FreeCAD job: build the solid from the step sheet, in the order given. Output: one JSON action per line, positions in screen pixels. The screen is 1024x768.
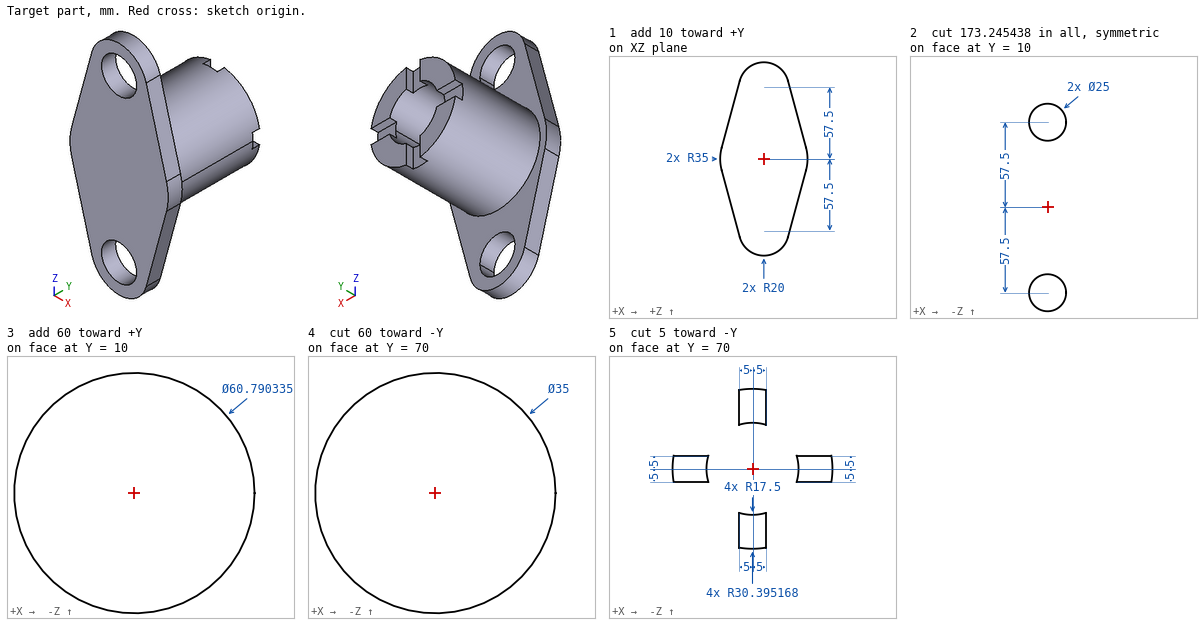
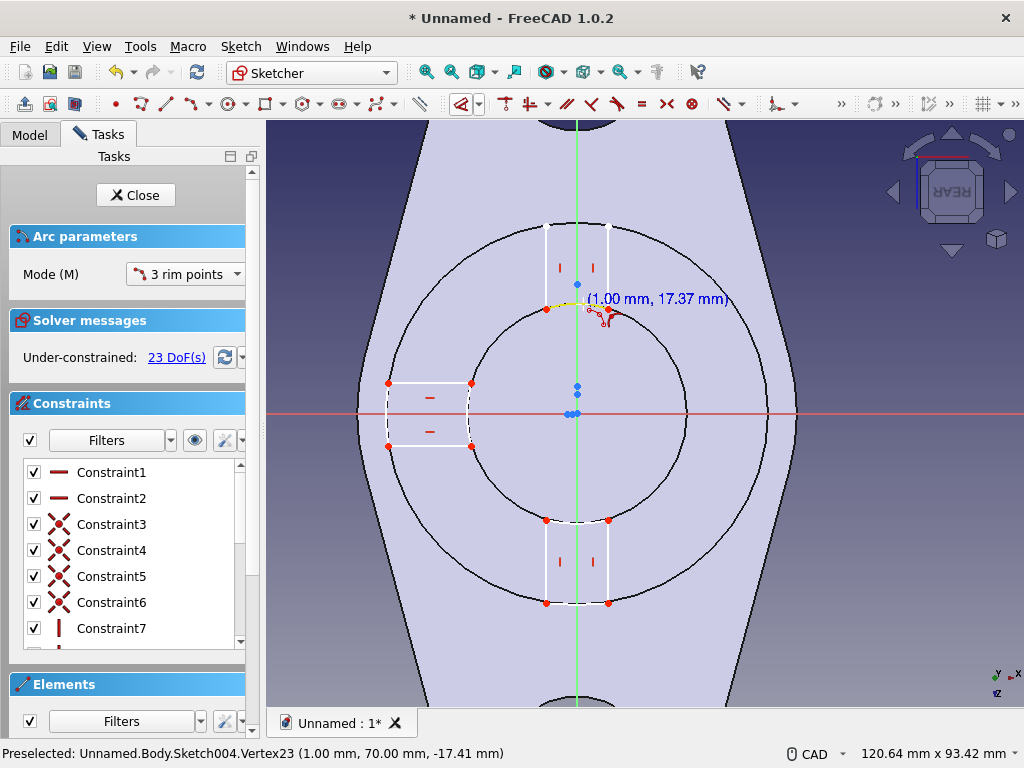
{"action": "left_click", "coordinate": [608, 226]}
{"action": "left_click", "coordinate": [546, 226]}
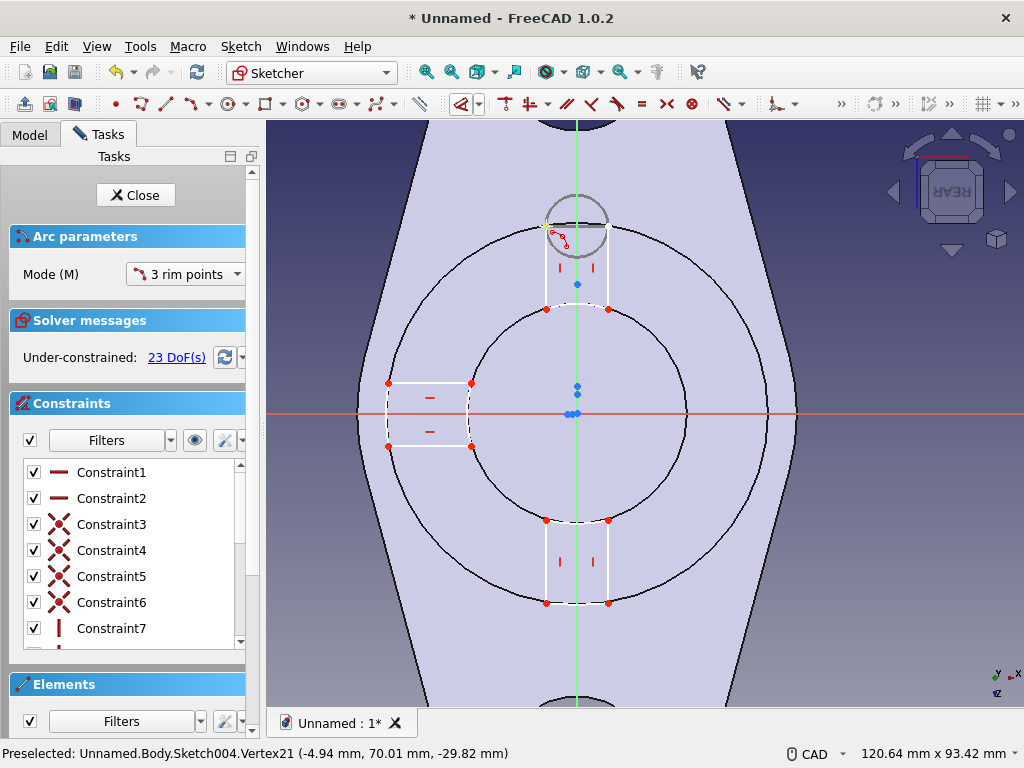
{"action": "scroll", "coordinate": [583, 223], "scroll_direction": "up", "scroll_amount": 10}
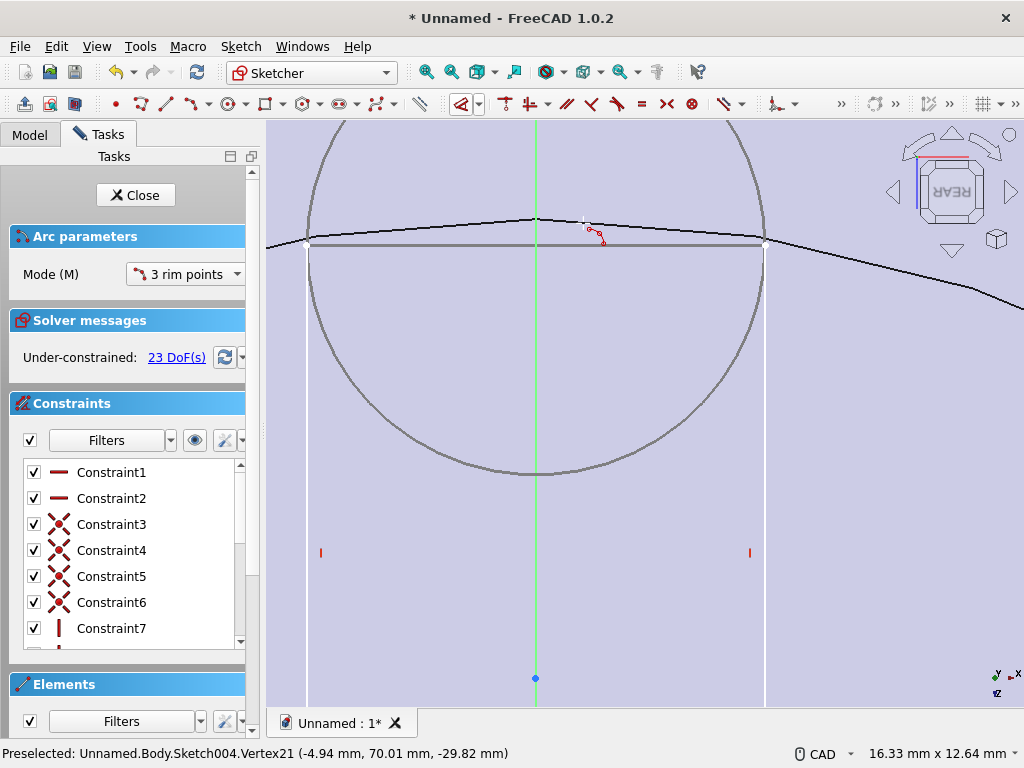
{"action": "left_click", "coordinate": [583, 220]}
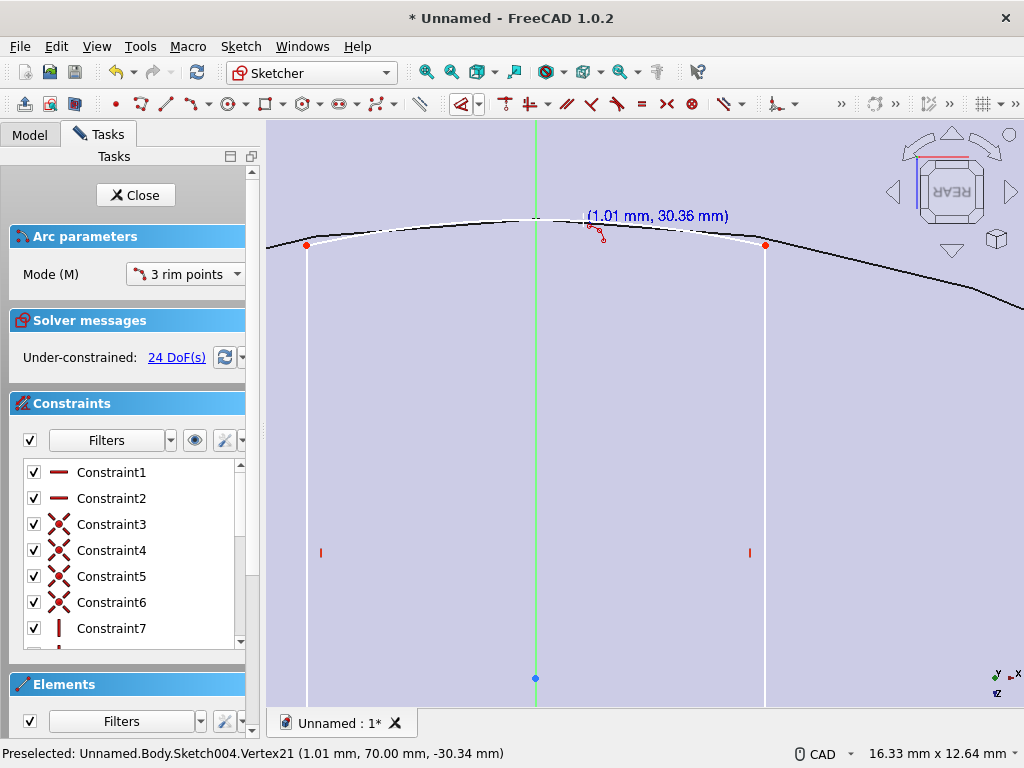
{"action": "key", "text": "g l"}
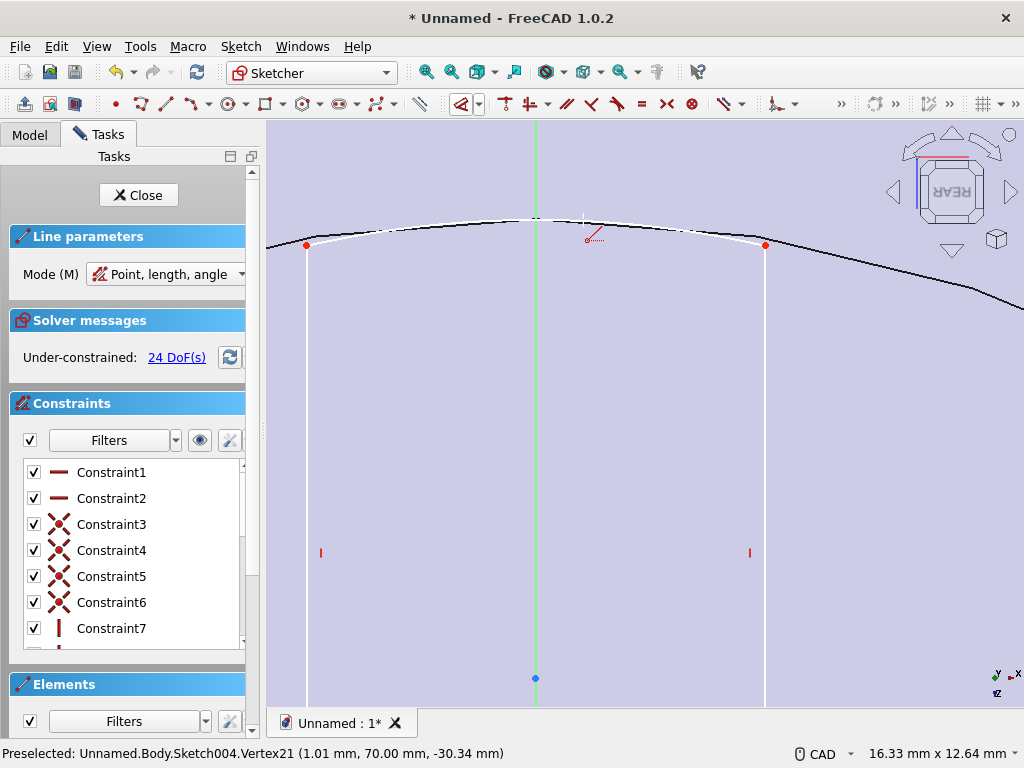
{"action": "scroll", "coordinate": [583, 223], "scroll_direction": "down", "scroll_amount": 10}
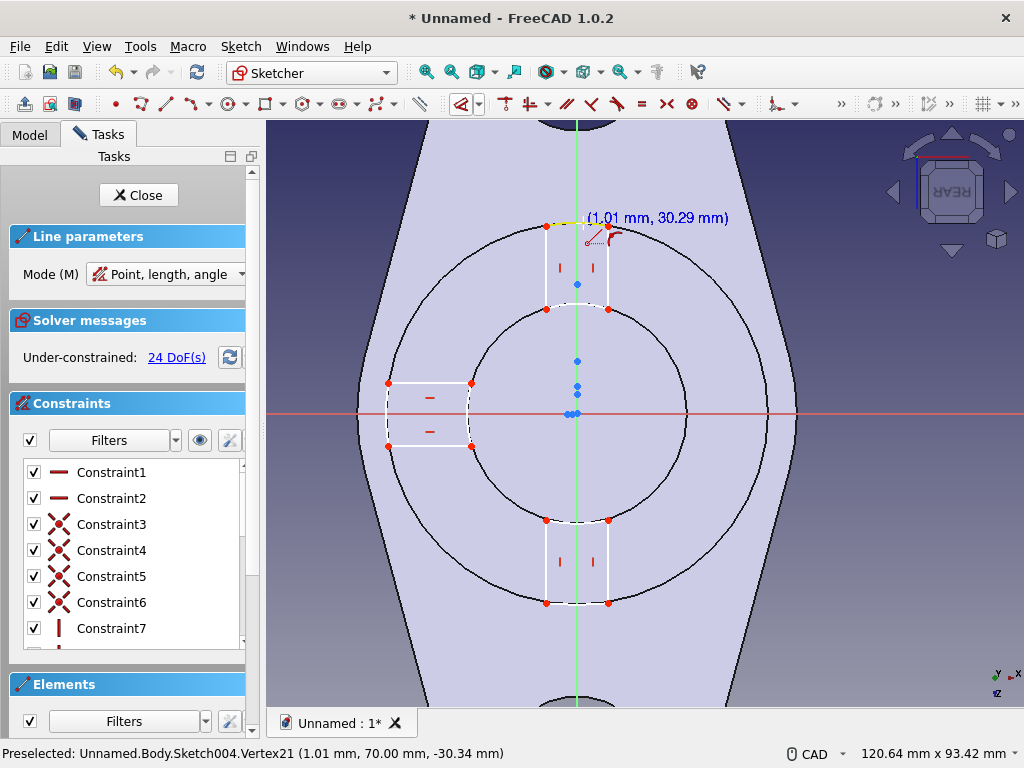
{"action": "left_click", "coordinate": [765, 382]}
{"action": "left_click", "coordinate": [682, 382]}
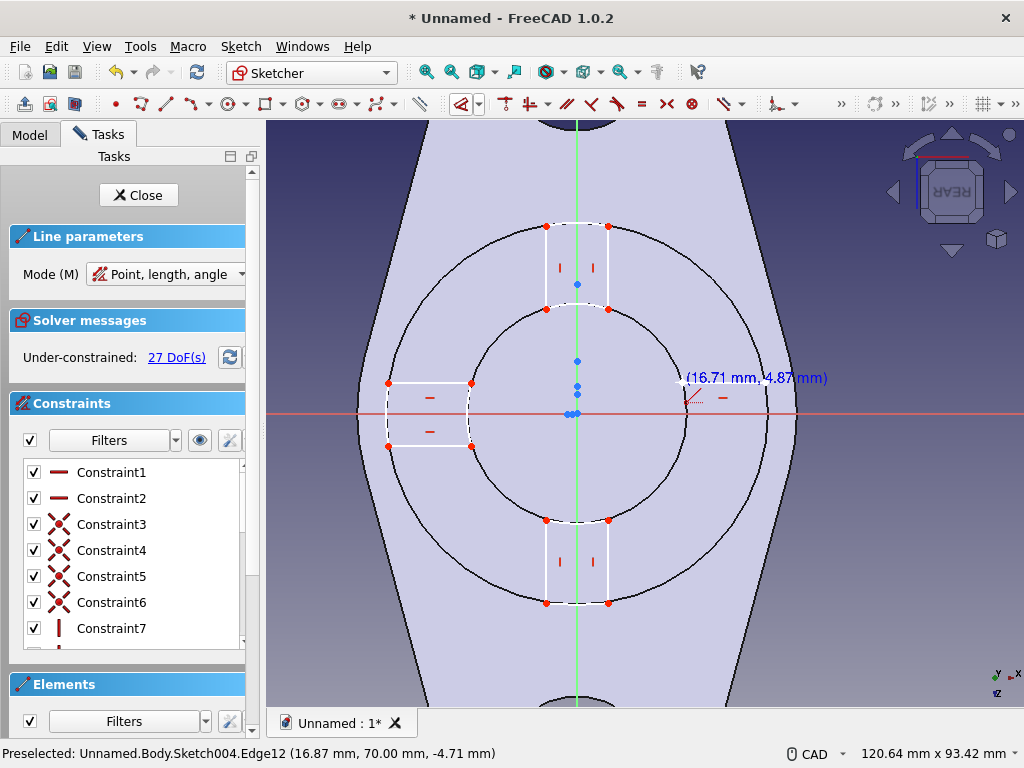
{"action": "left_click", "coordinate": [682, 445]}
{"action": "left_click", "coordinate": [765, 445]}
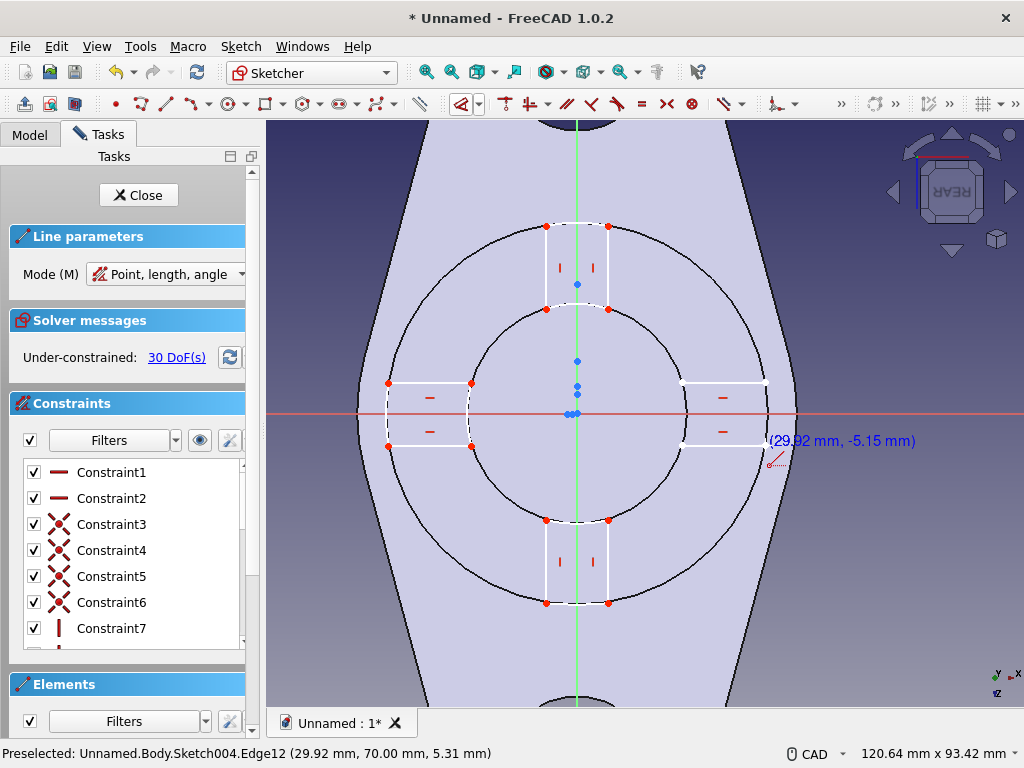
{"action": "left_click", "coordinate": [190, 104]}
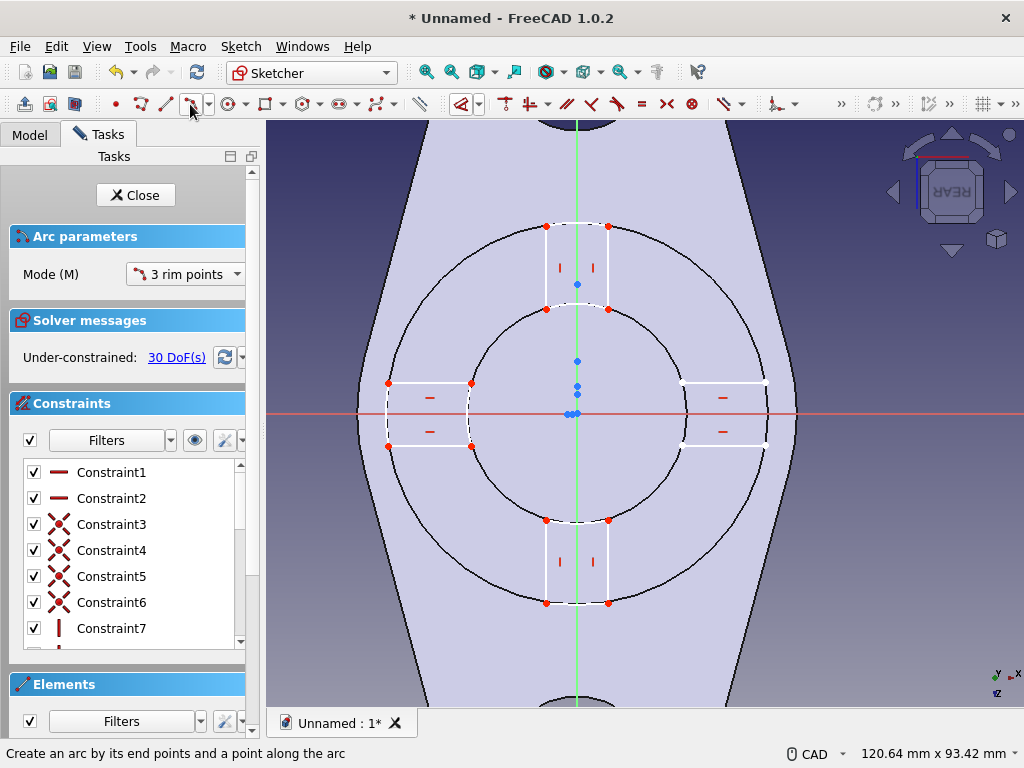
{"action": "left_click", "coordinate": [682, 383]}
{"action": "left_click", "coordinate": [682, 446]}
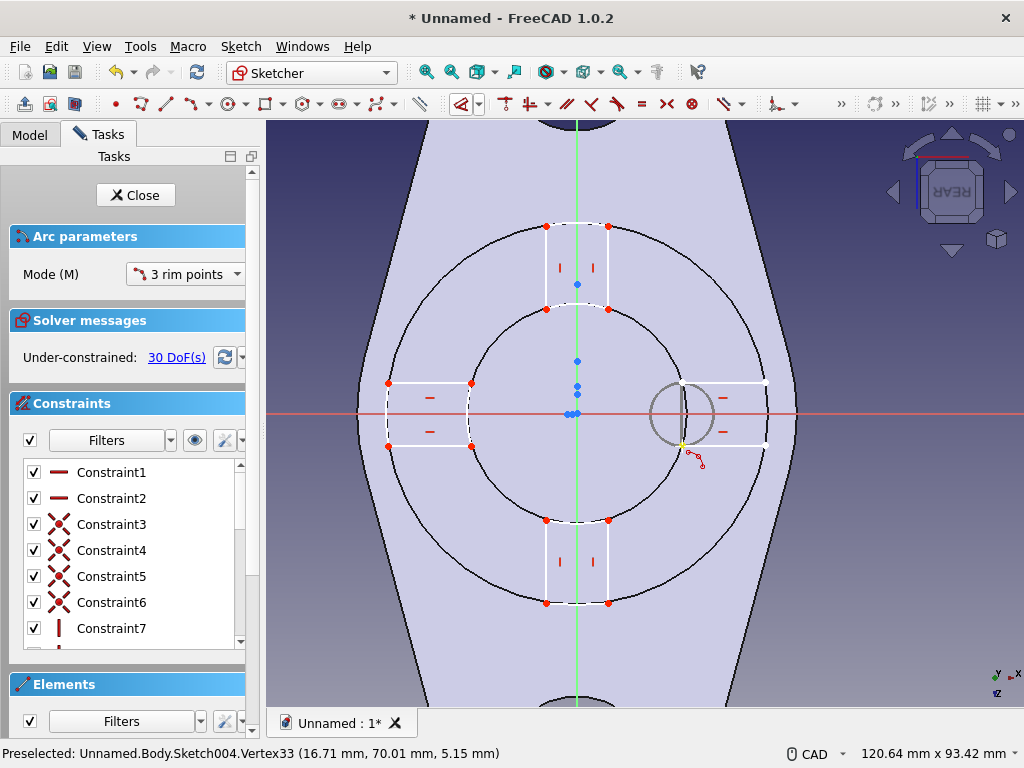
{"action": "scroll", "coordinate": [687, 420], "scroll_direction": "up", "scroll_amount": 7}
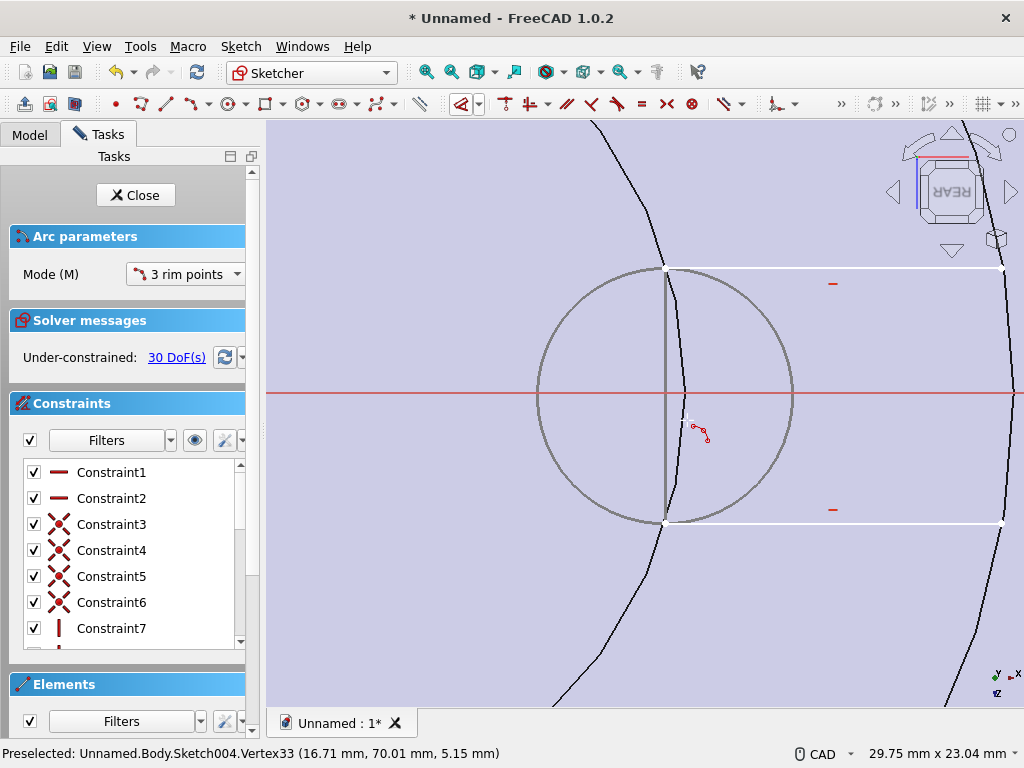
{"action": "left_click", "coordinate": [684, 418]}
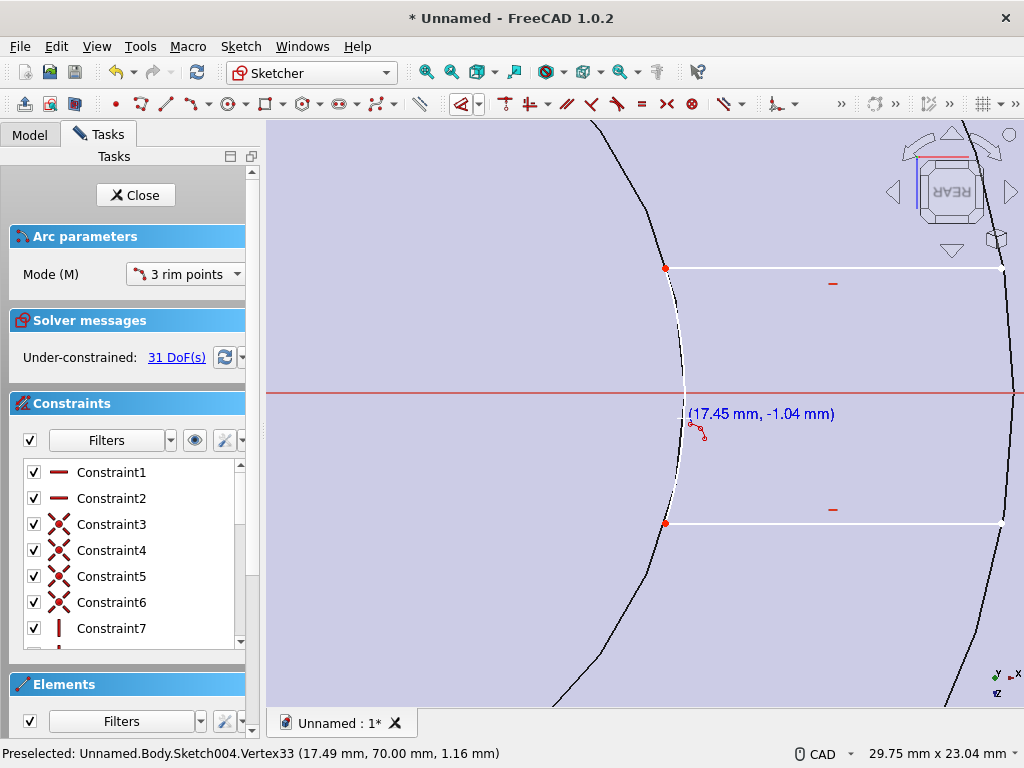
{"action": "scroll", "coordinate": [687, 420], "scroll_direction": "down", "scroll_amount": 7}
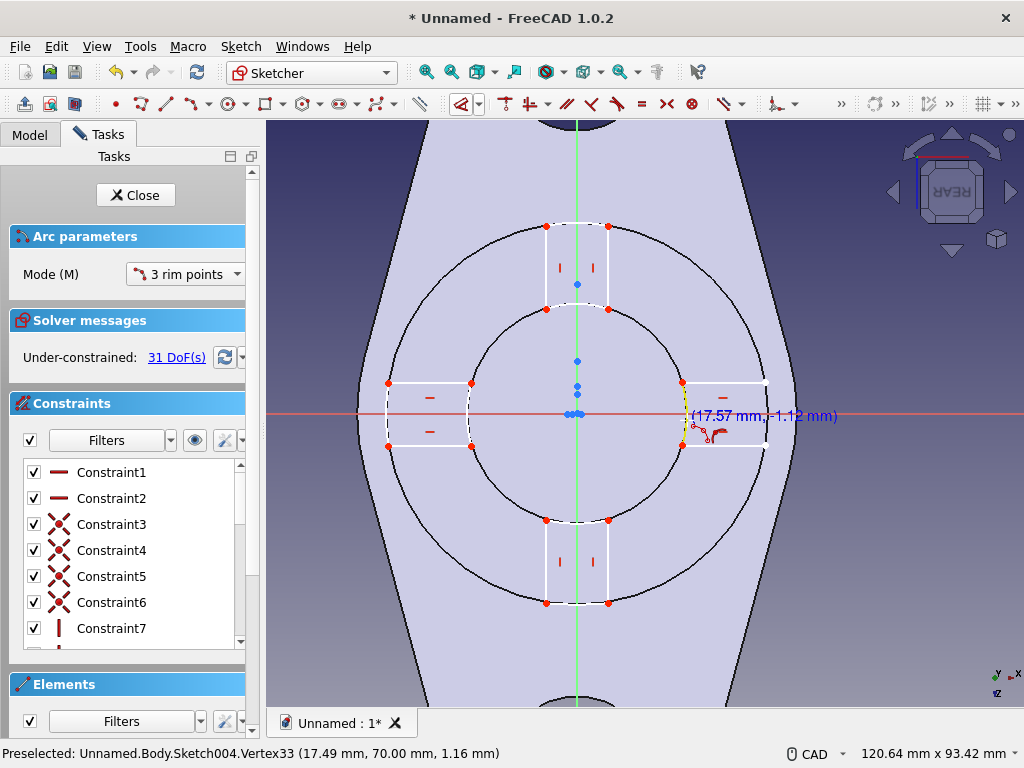
{"action": "left_click", "coordinate": [765, 446]}
{"action": "left_click", "coordinate": [765, 383]}